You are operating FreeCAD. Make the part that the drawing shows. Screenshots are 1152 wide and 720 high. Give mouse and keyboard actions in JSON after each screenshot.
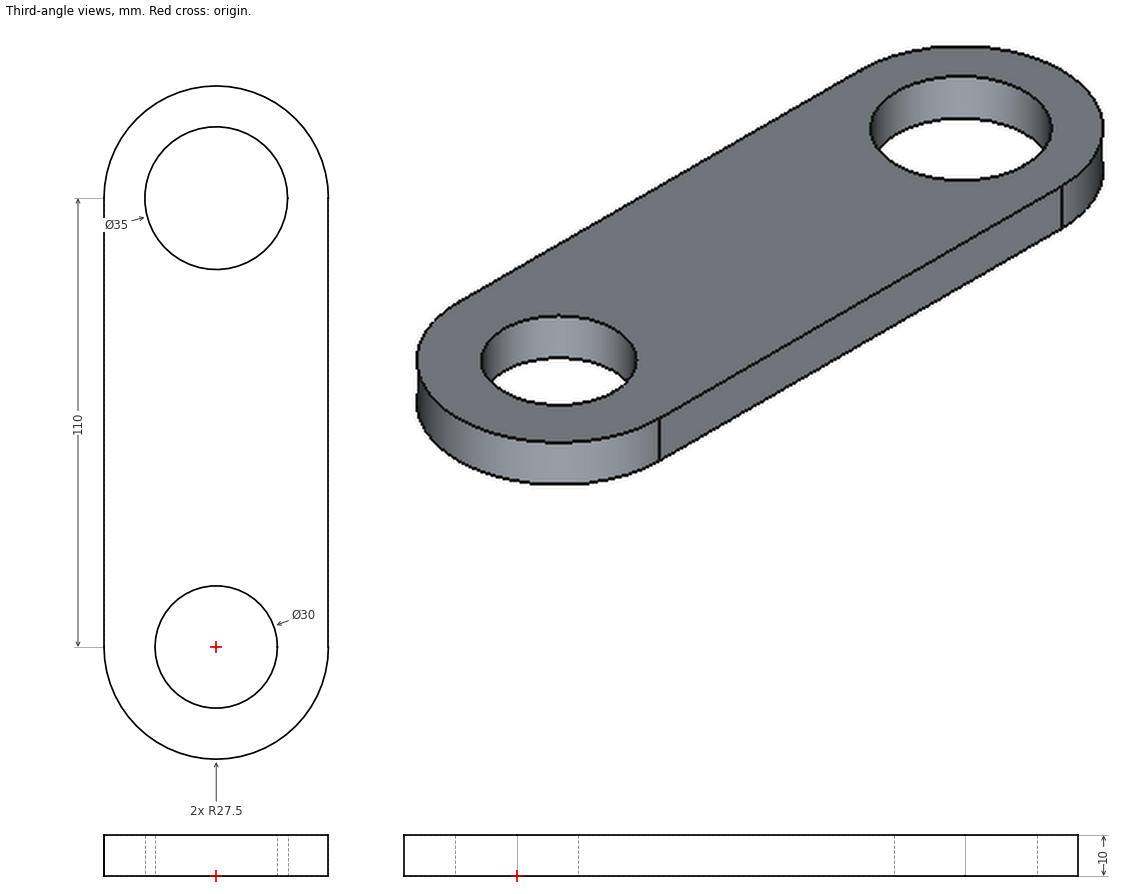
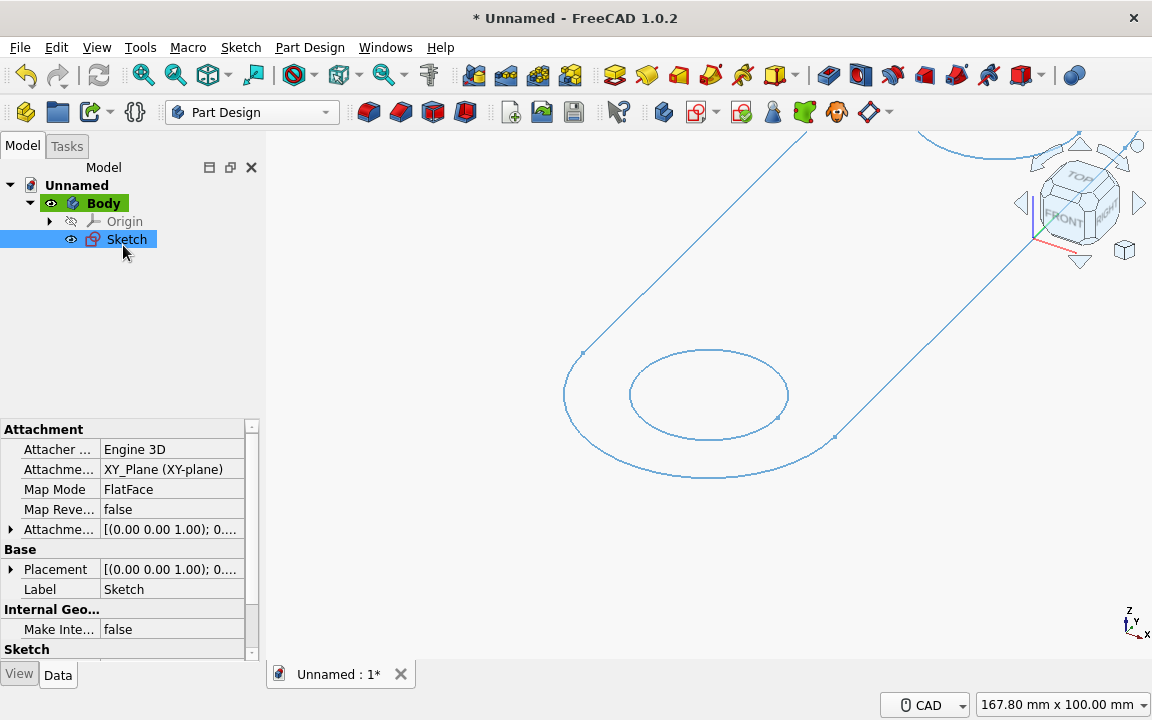
{"action": "left_click", "coordinate": [616, 76]}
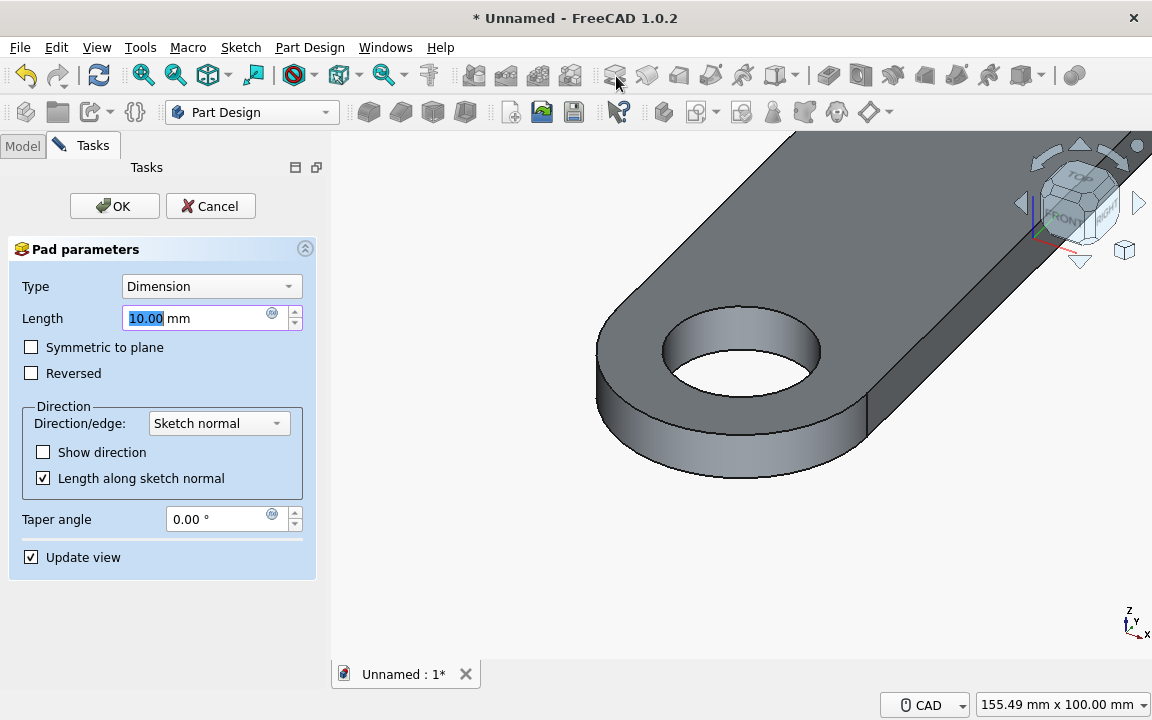
{"action": "type", "text": "10"}
{"action": "key", "text": "Tab"}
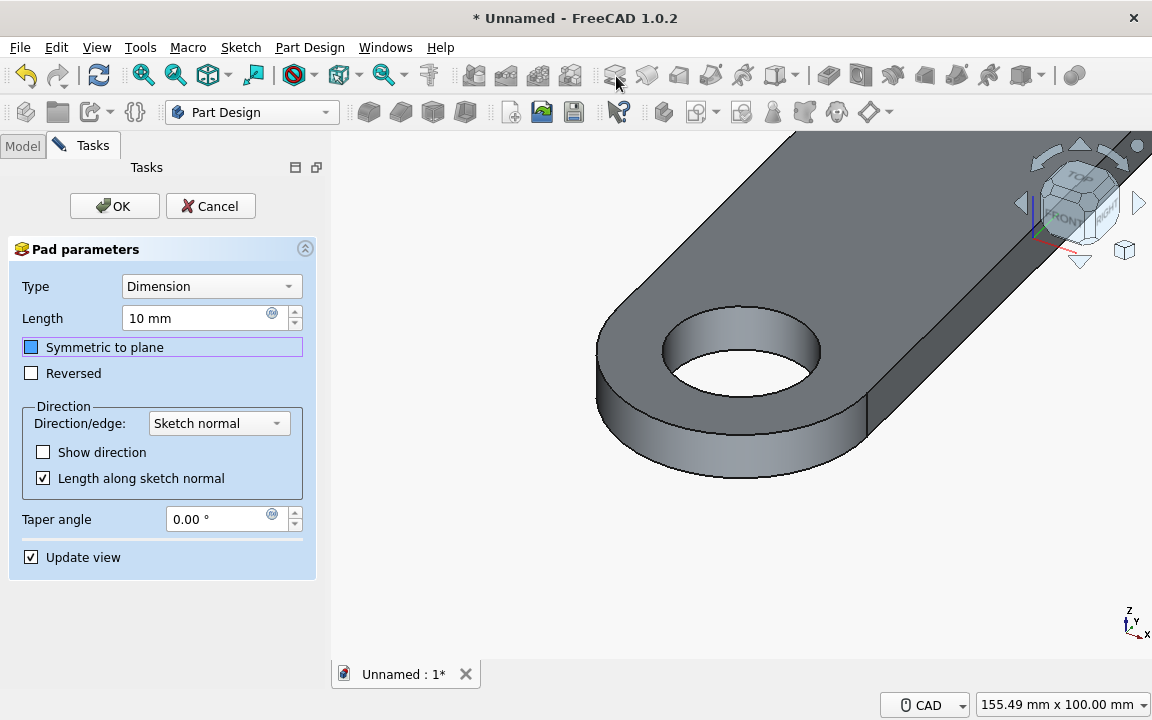
{"action": "left_click", "coordinate": [115, 206]}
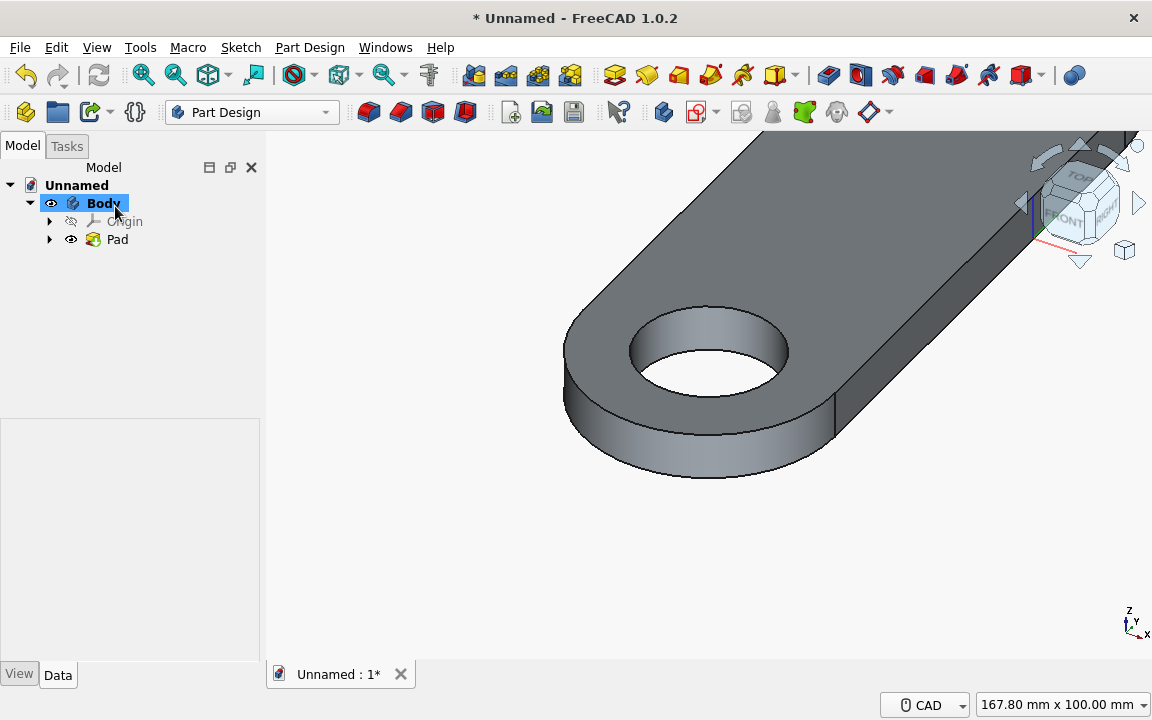
{"action": "key", "text": "0"}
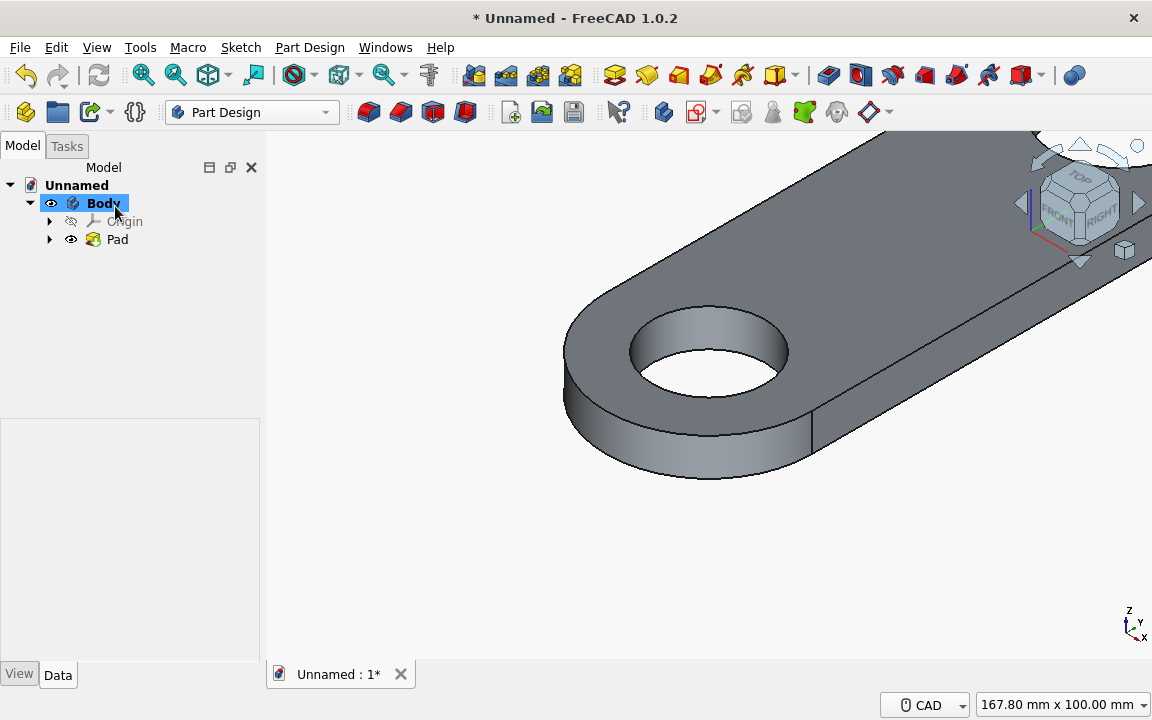
{"action": "key", "text": "v f"}